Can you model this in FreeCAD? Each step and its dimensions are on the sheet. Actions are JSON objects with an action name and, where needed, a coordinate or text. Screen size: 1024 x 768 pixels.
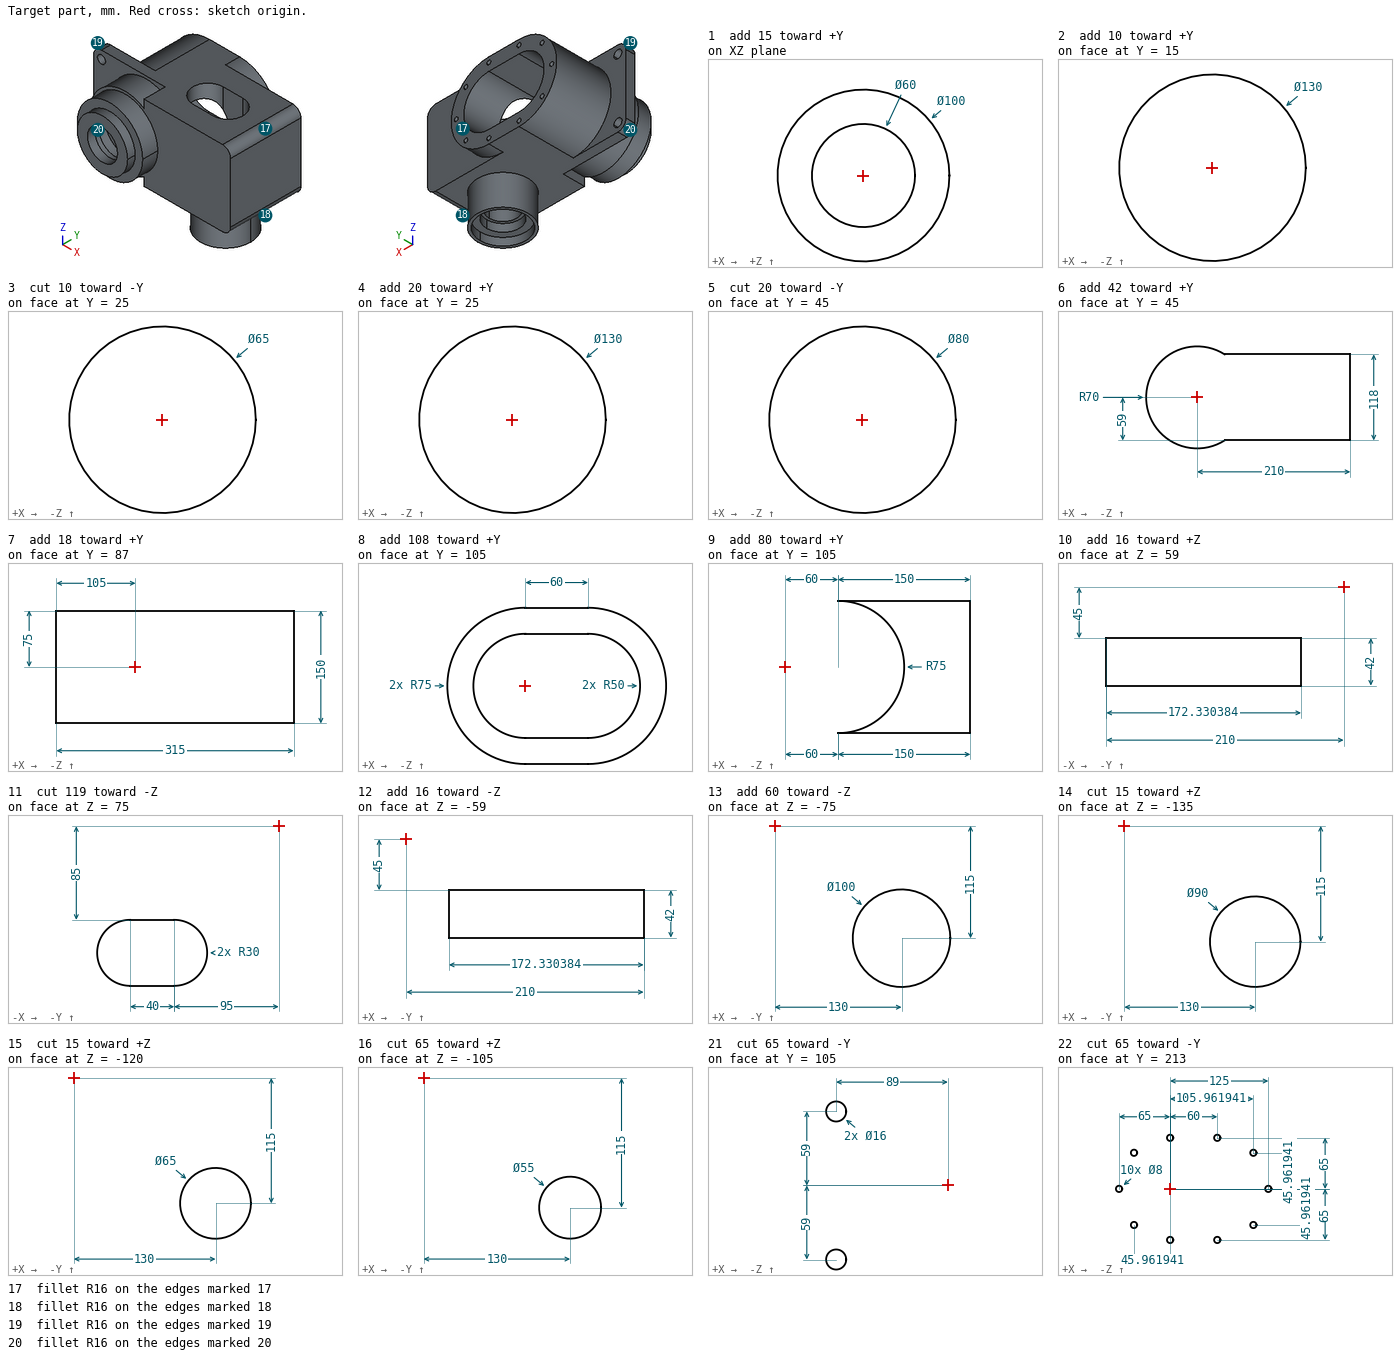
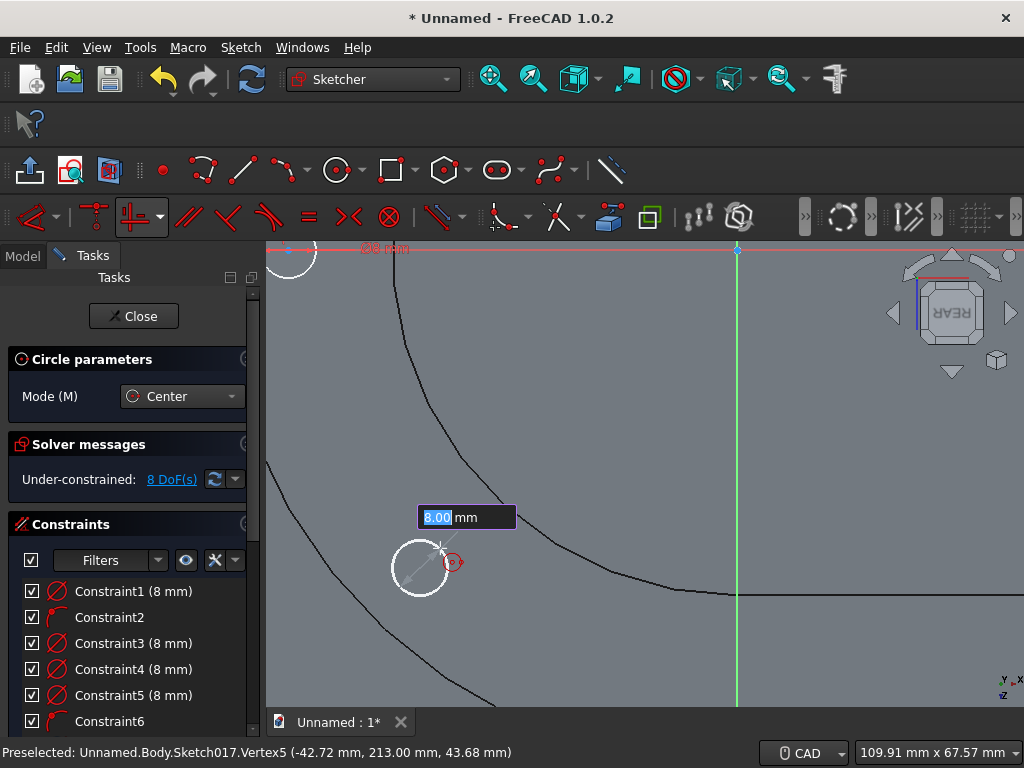
{"action": "type", "text": "8"}
{"action": "key", "text": "Return"}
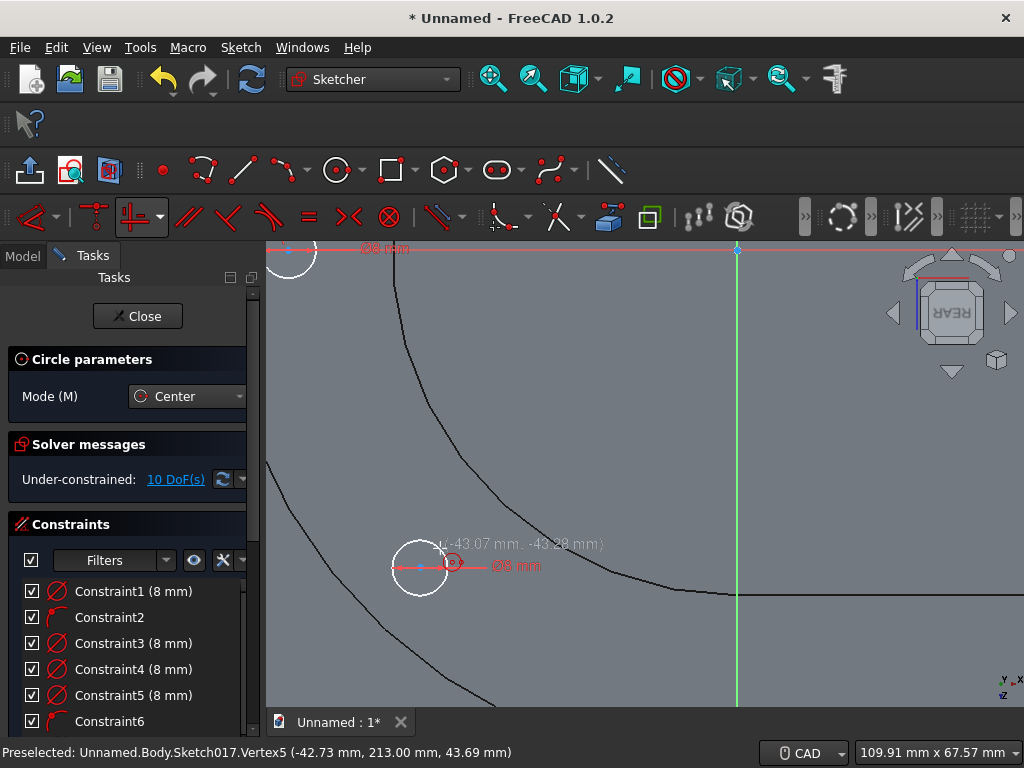
{"action": "scroll", "coordinate": [418, 570], "scroll_direction": "down", "scroll_amount": 6}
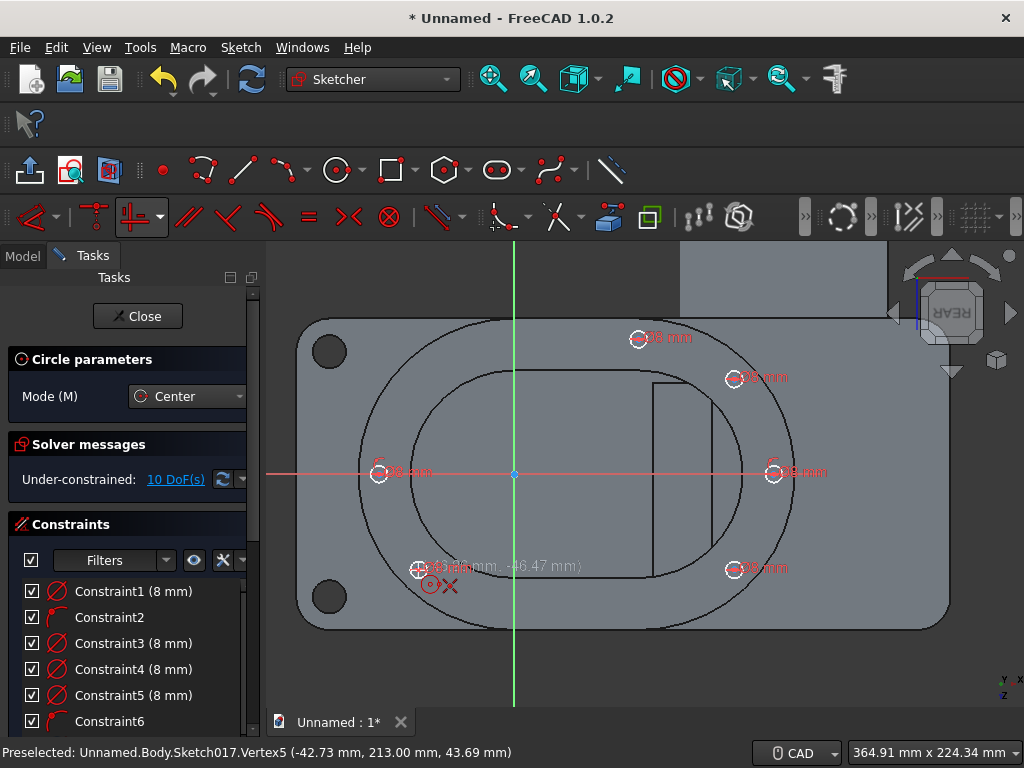
{"action": "scroll", "coordinate": [419, 379], "scroll_direction": "up", "scroll_amount": 6}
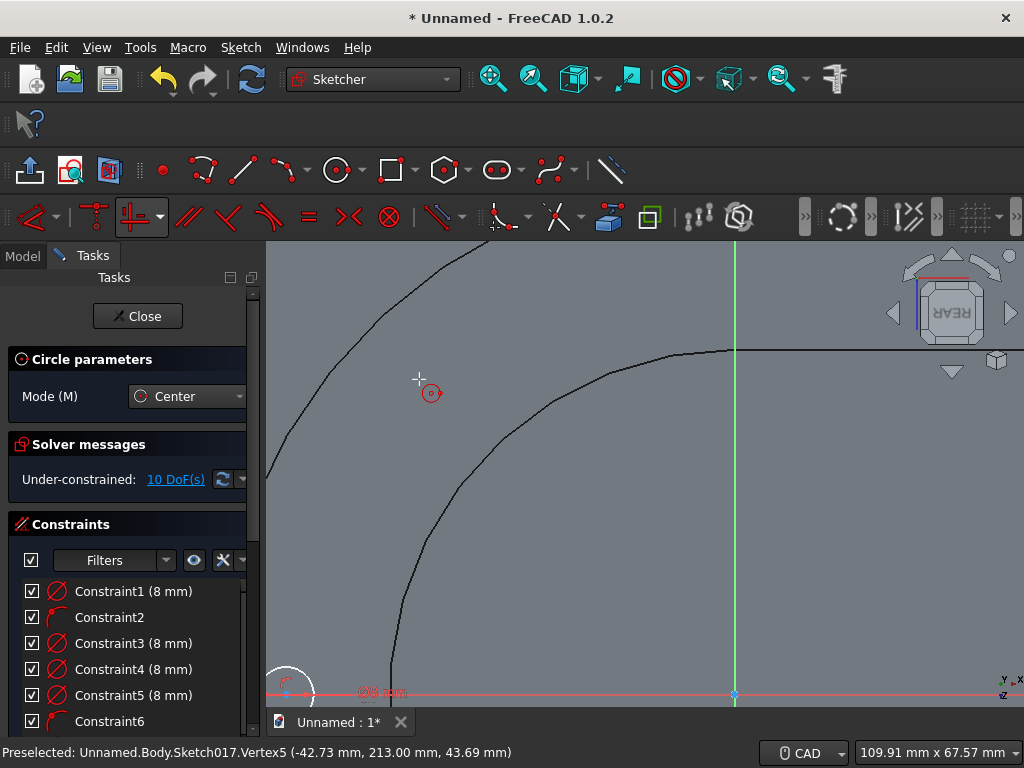
{"action": "left_click", "coordinate": [418, 378]}
{"action": "mouse_move", "coordinate": [437, 358]}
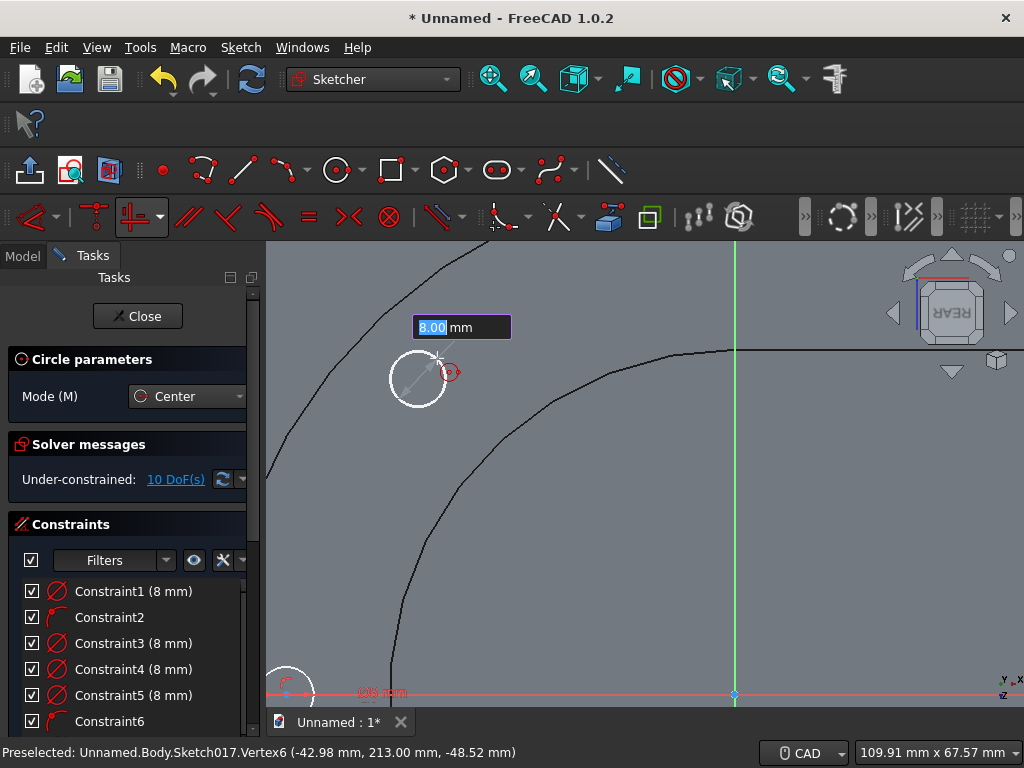
{"action": "type", "text": "8"}
{"action": "key", "text": "Return"}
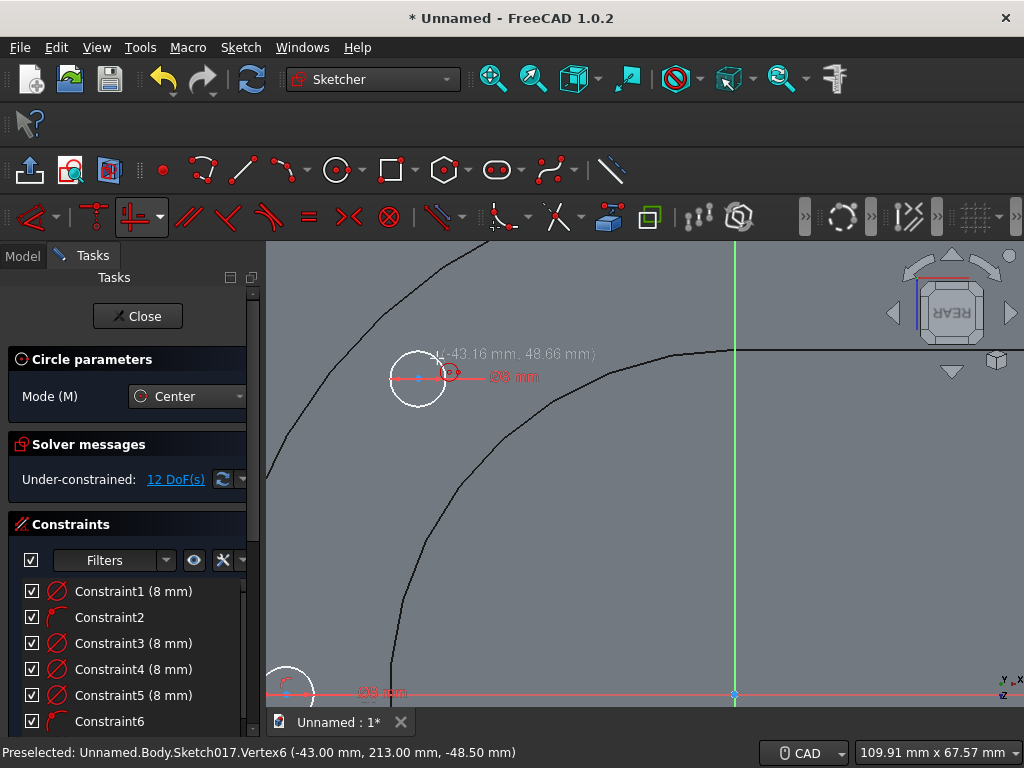
{"action": "scroll", "coordinate": [419, 379], "scroll_direction": "down", "scroll_amount": 6}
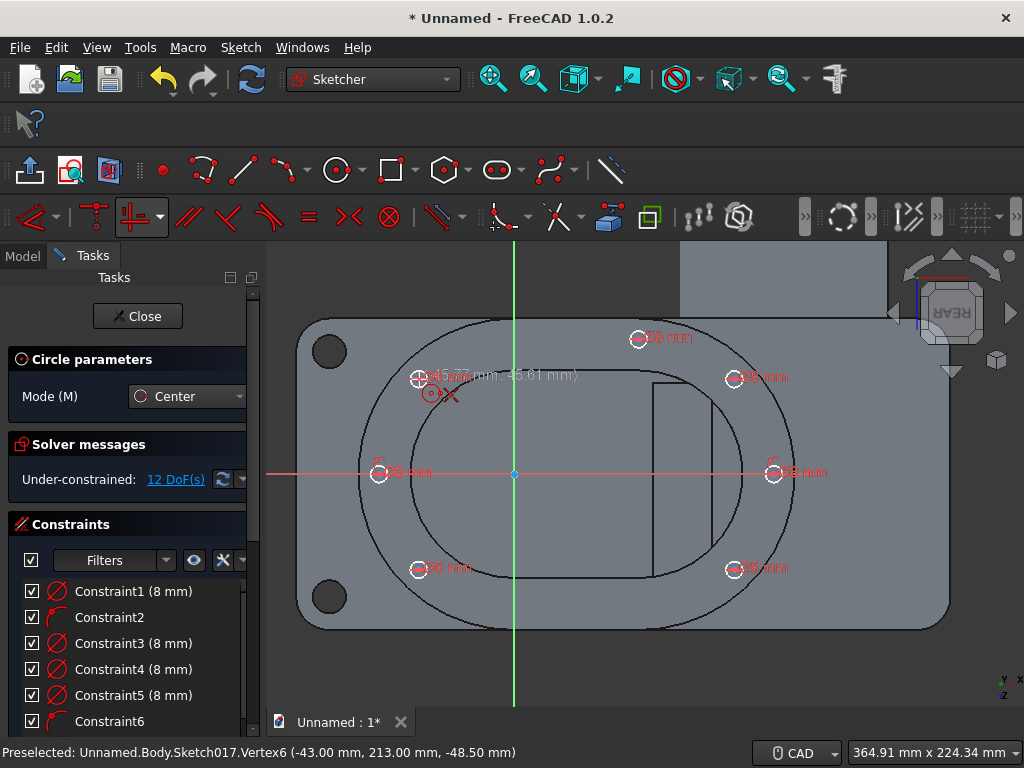
{"action": "scroll", "coordinate": [514, 339], "scroll_direction": "up", "scroll_amount": 6}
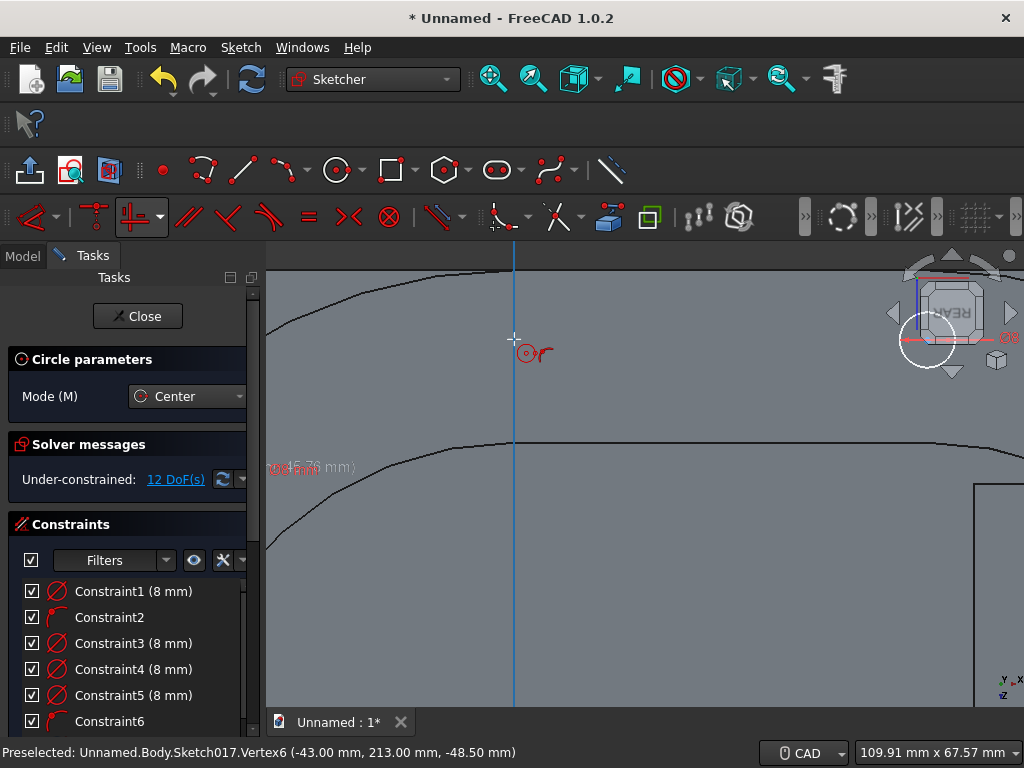
{"action": "left_click", "coordinate": [514, 339]}
{"action": "mouse_move", "coordinate": [533, 320]}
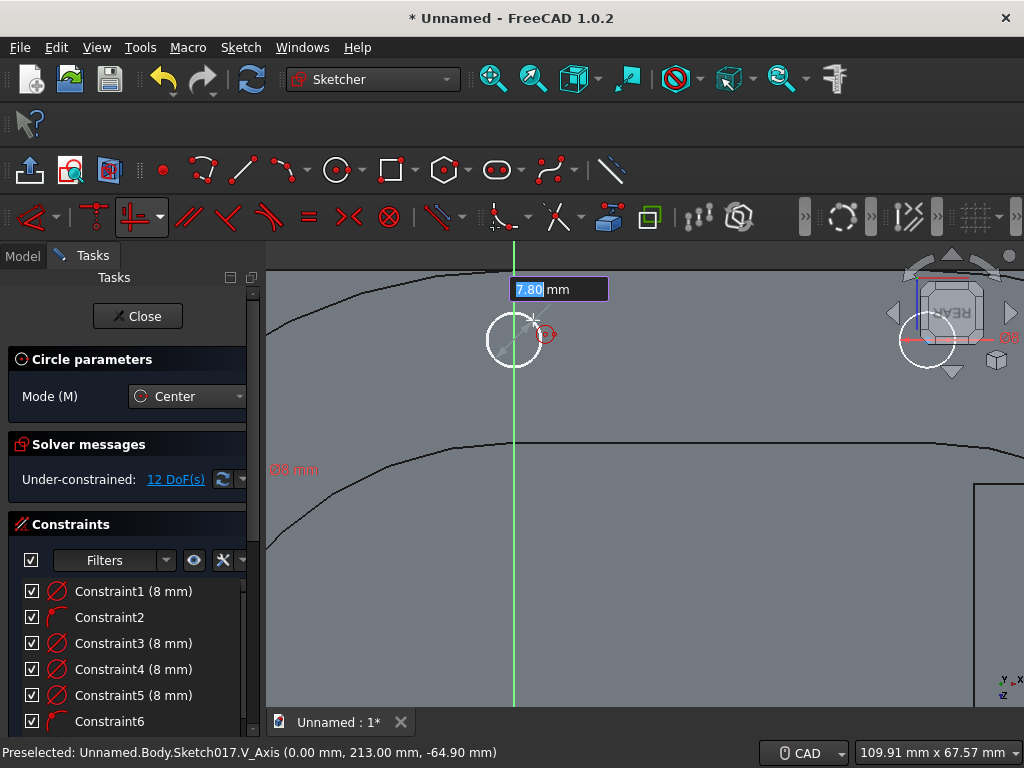
{"action": "type", "text": "8"}
{"action": "key", "text": "Return"}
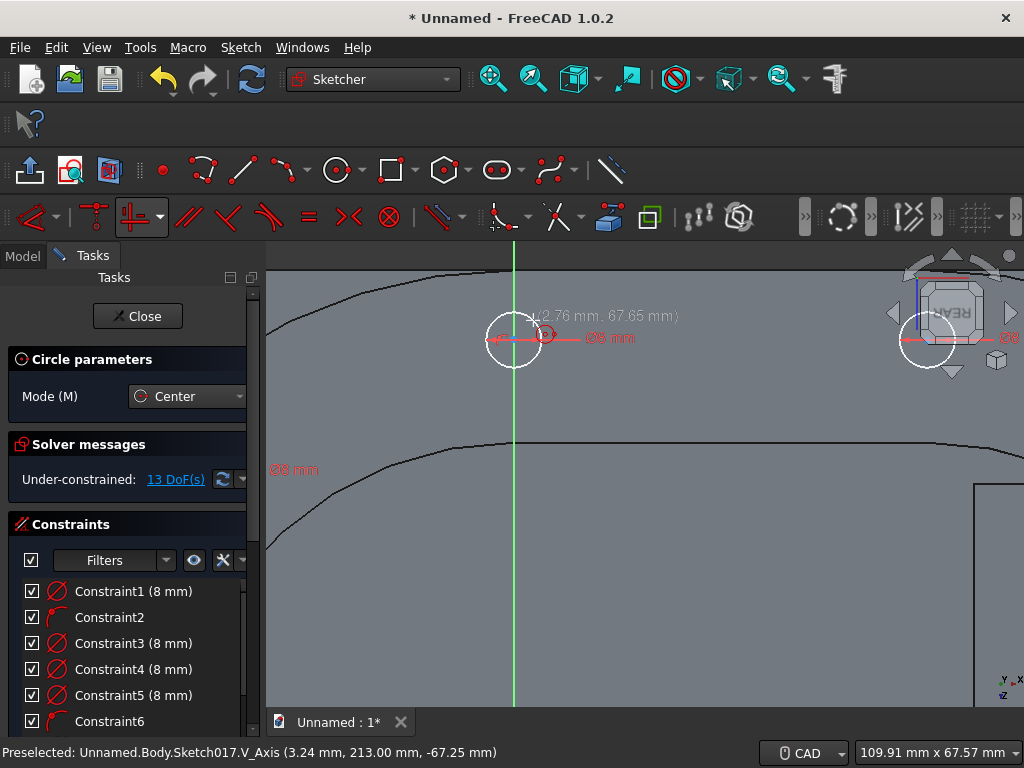
{"action": "scroll", "coordinate": [514, 339], "scroll_direction": "down", "scroll_amount": 6}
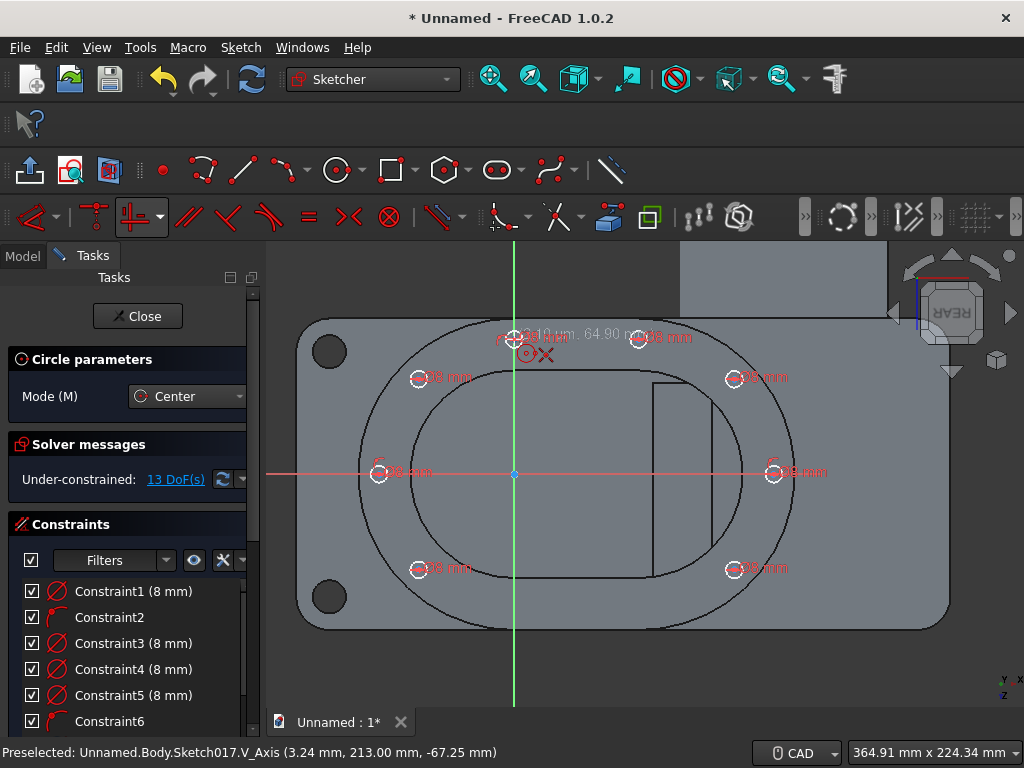
{"action": "scroll", "coordinate": [639, 609], "scroll_direction": "up", "scroll_amount": 6}